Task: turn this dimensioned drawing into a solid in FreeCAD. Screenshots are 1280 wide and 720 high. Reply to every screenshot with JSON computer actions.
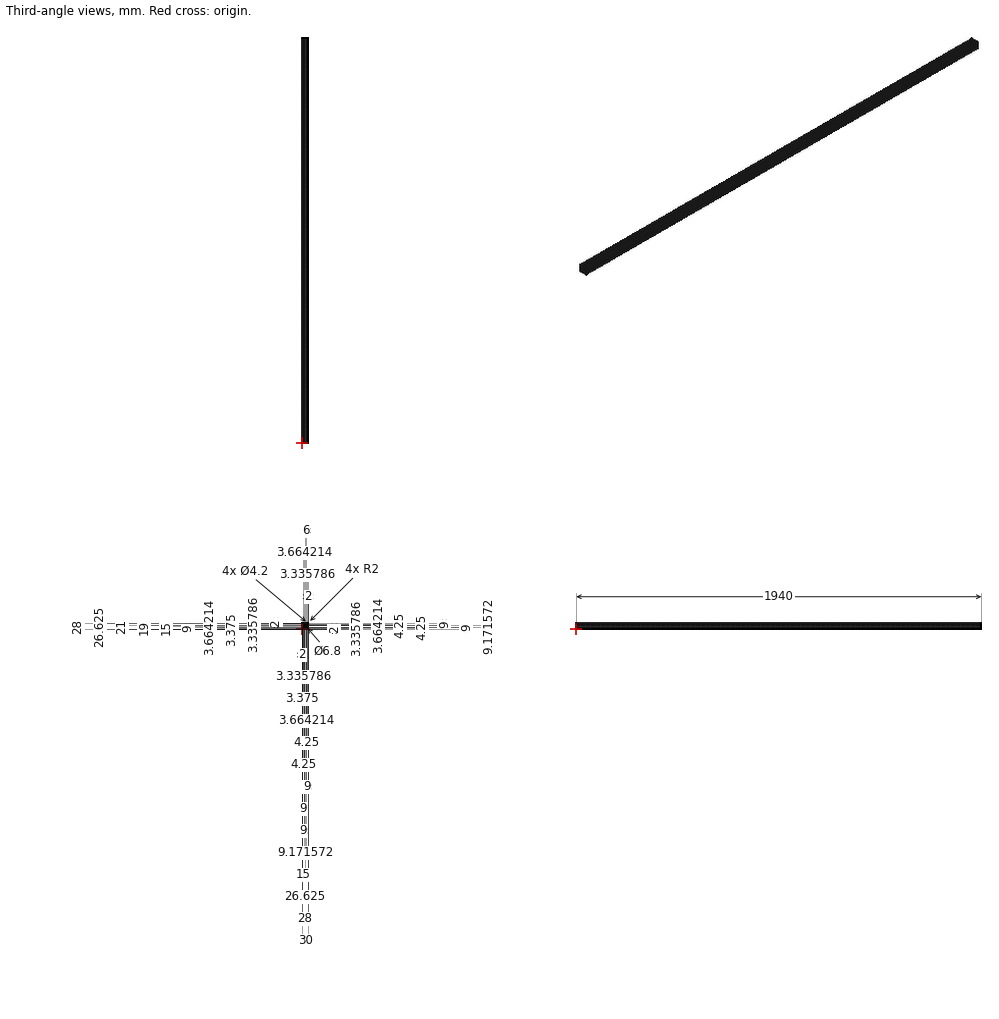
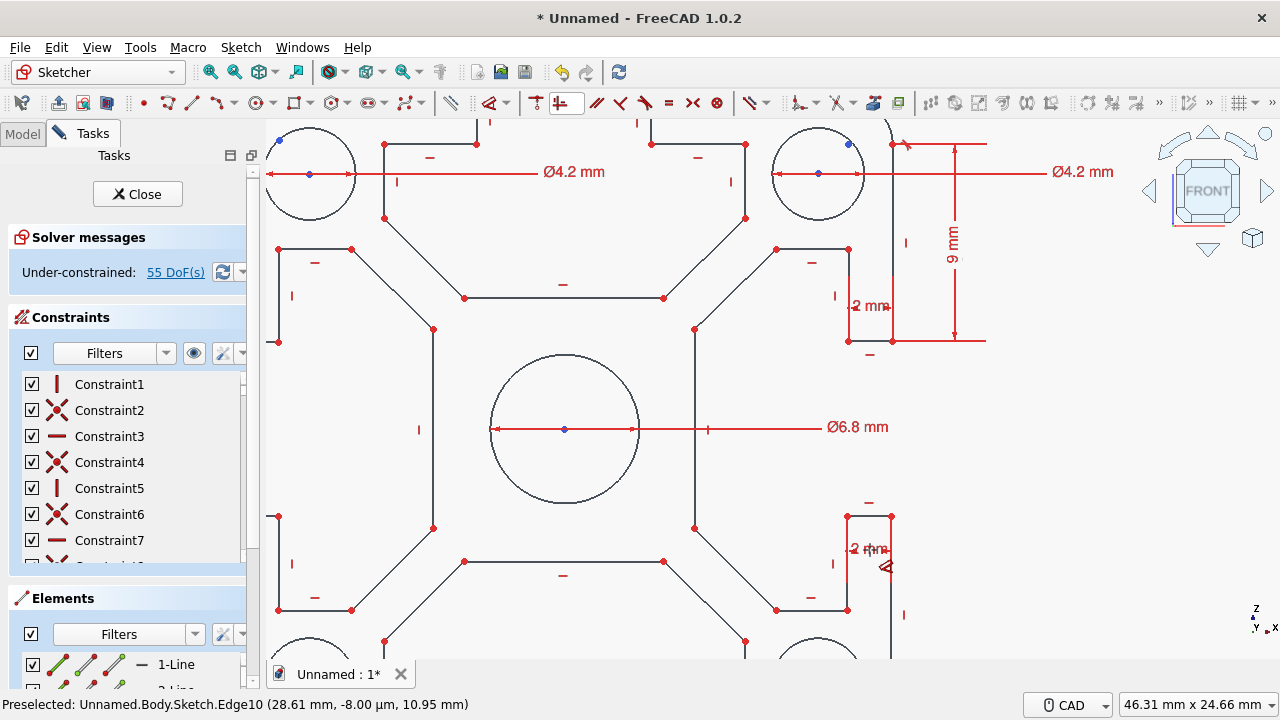
{"action": "left_click", "coordinate": [891, 575]}
{"action": "left_click", "coordinate": [925, 574]}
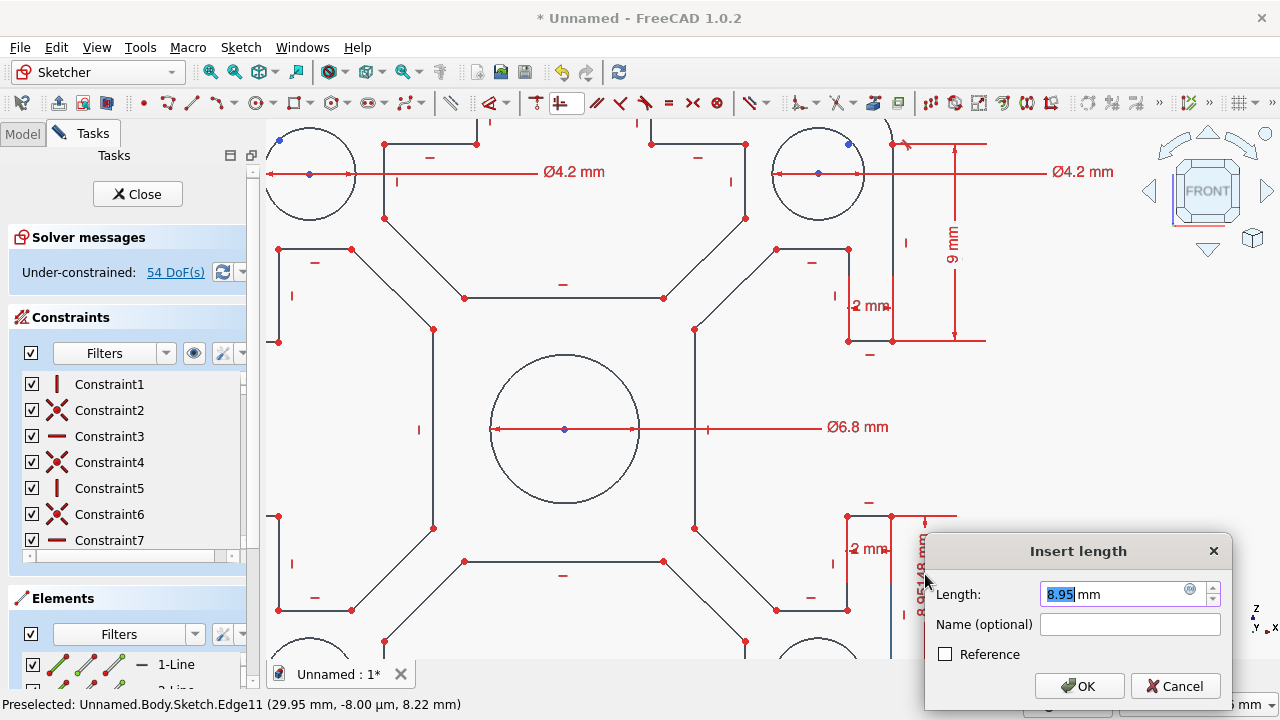
{"action": "type", "text": "9"}
{"action": "key", "text": "Return"}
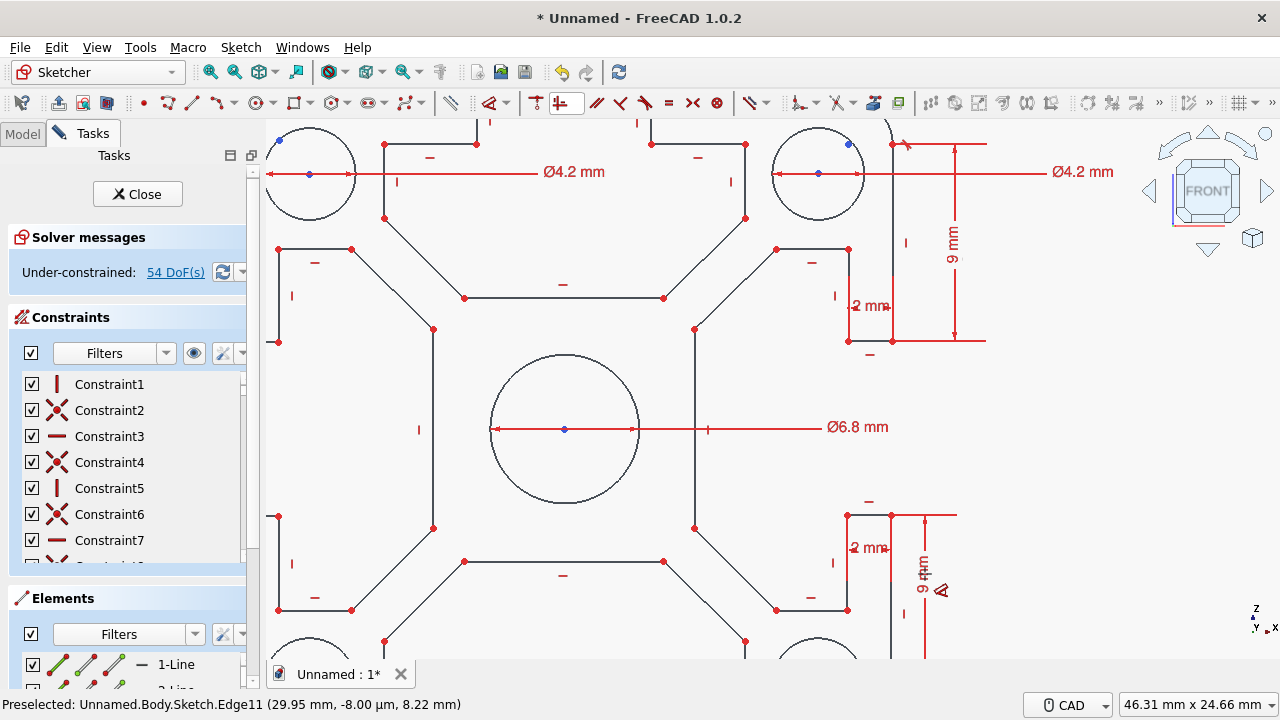
{"action": "scroll", "coordinate": [875, 342], "scroll_direction": "down", "scroll_amount": 3}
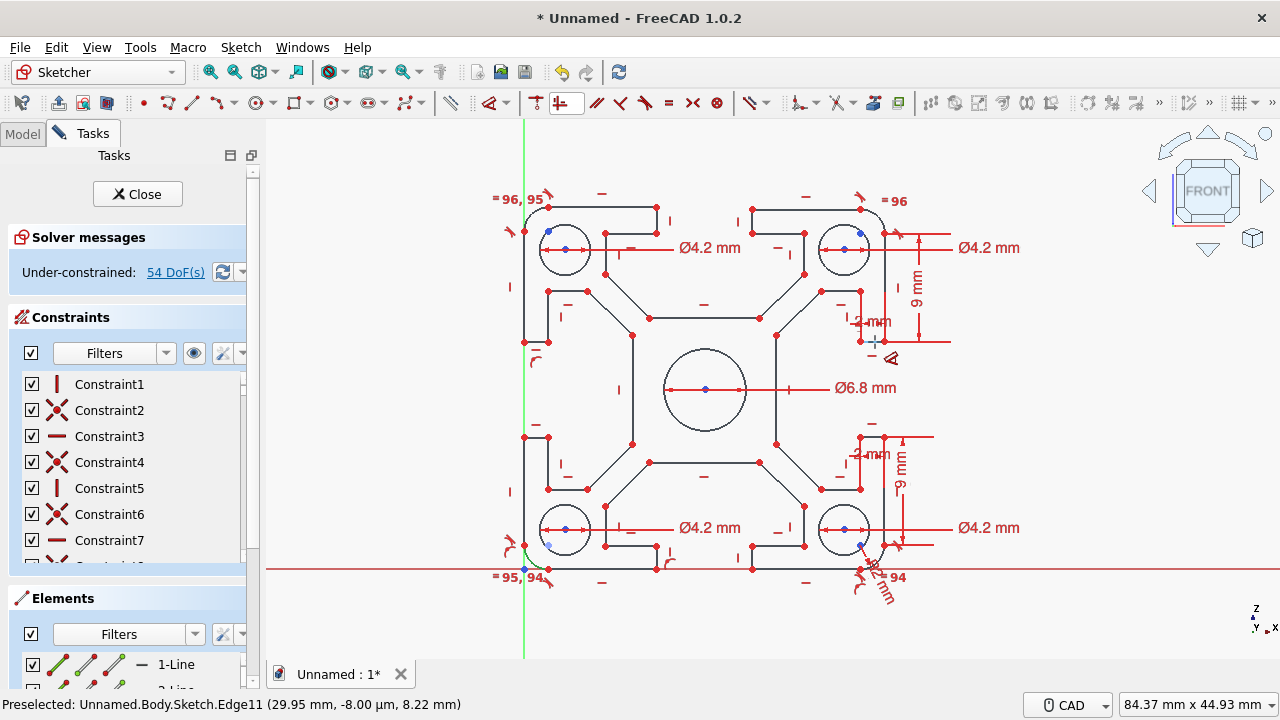
{"action": "left_click", "coordinate": [828, 569]}
{"action": "left_click", "coordinate": [806, 603]}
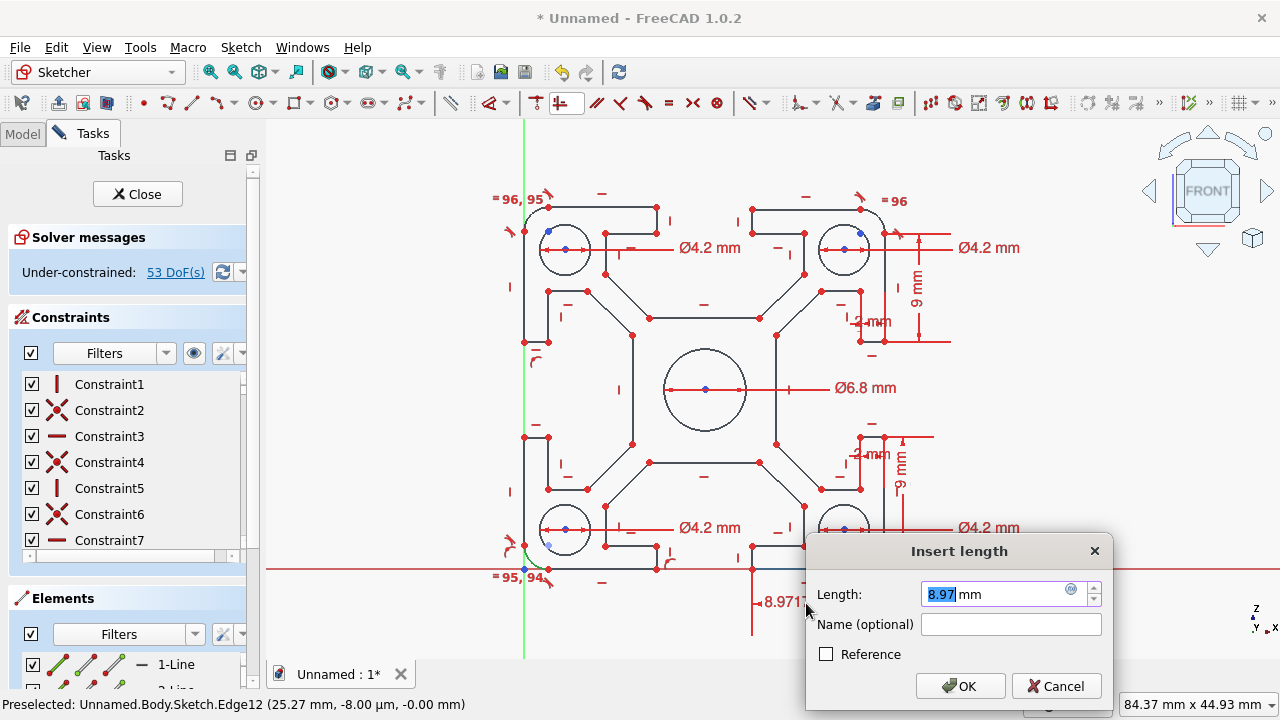
{"action": "type", "text": "9"}
{"action": "key", "text": "Return"}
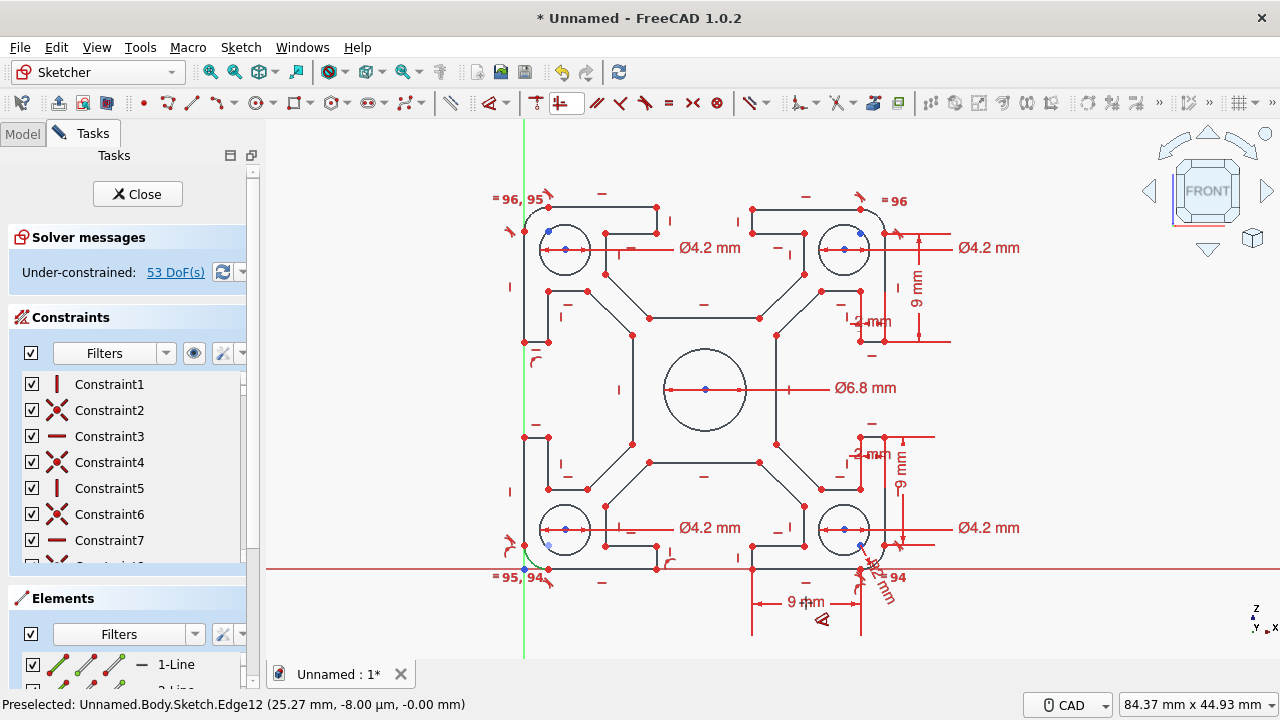
{"action": "scroll", "coordinate": [752, 560], "scroll_direction": "up", "scroll_amount": 3}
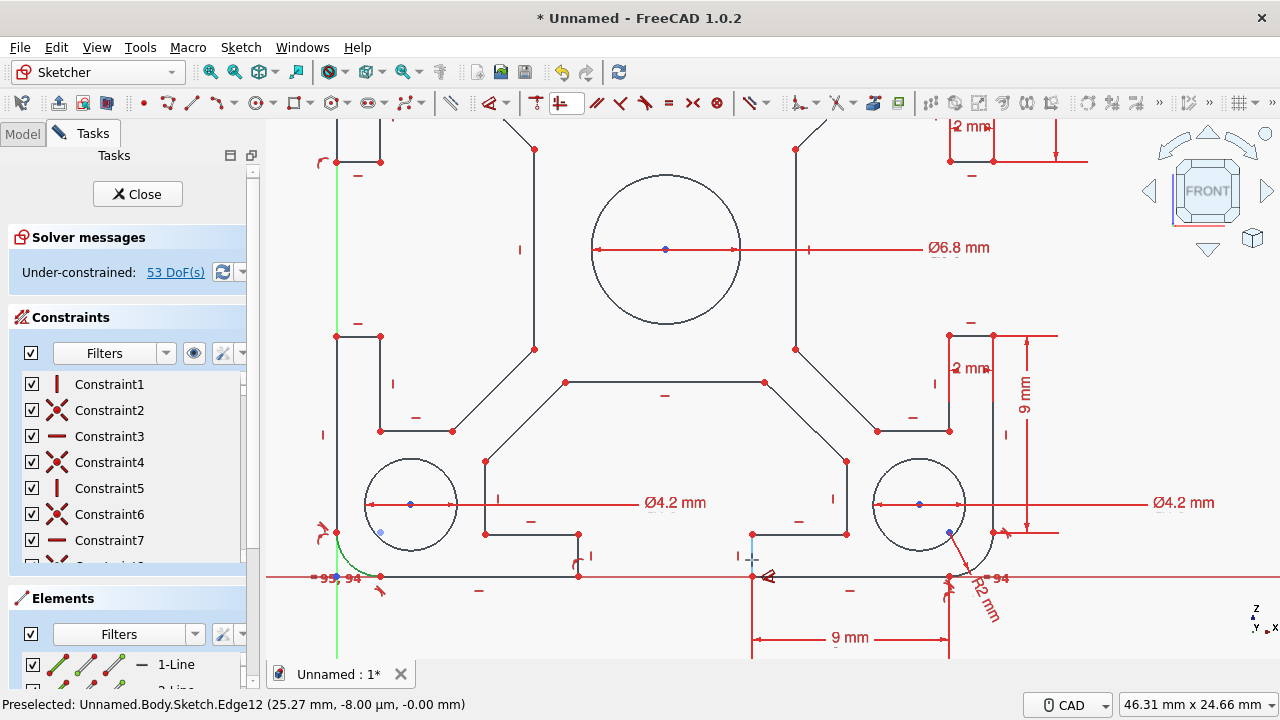
{"action": "left_click", "coordinate": [752, 560]}
{"action": "left_click", "coordinate": [786, 556]}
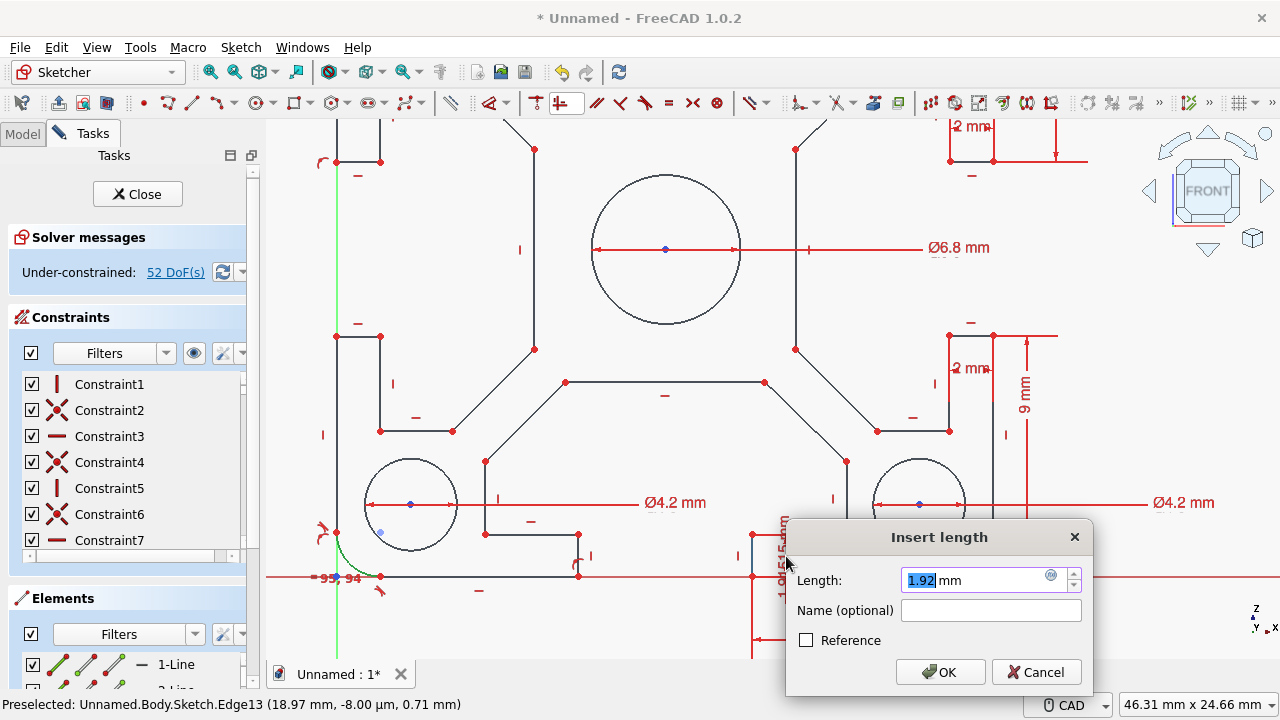
{"action": "type", "text": "2"}
{"action": "key", "text": "Return"}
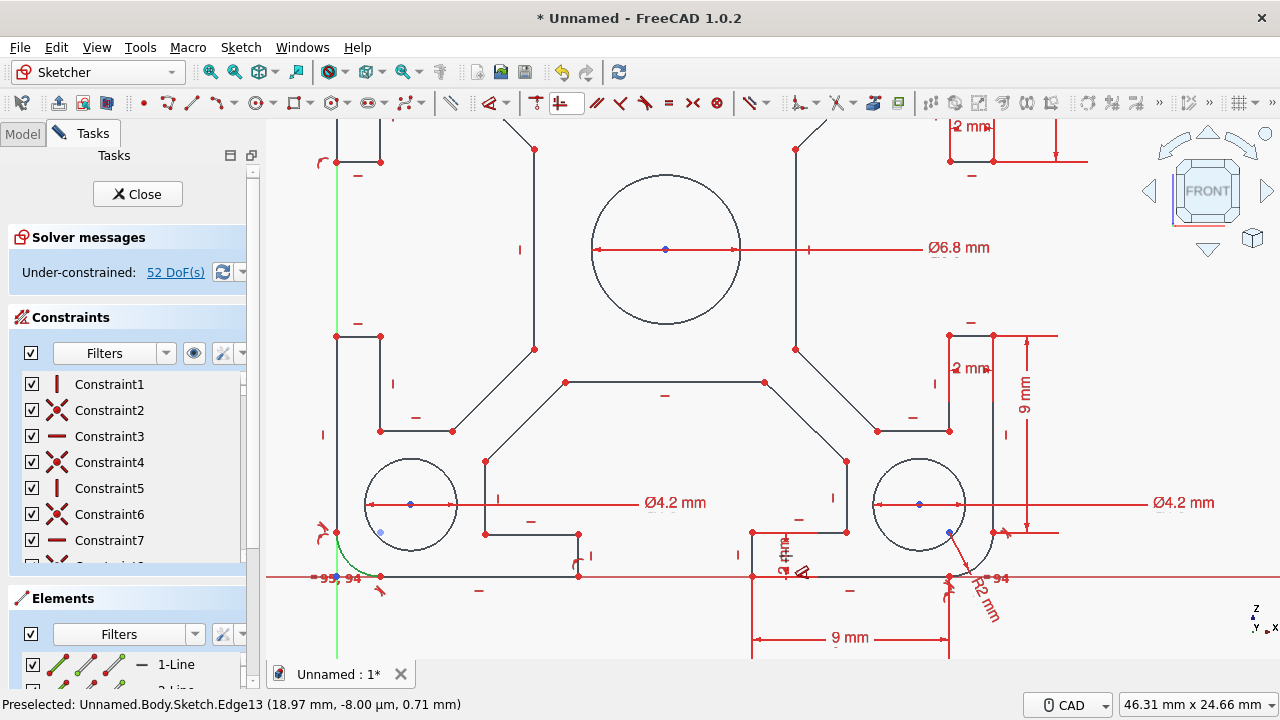
{"action": "left_click", "coordinate": [578, 547]}
{"action": "left_click", "coordinate": [544, 556]}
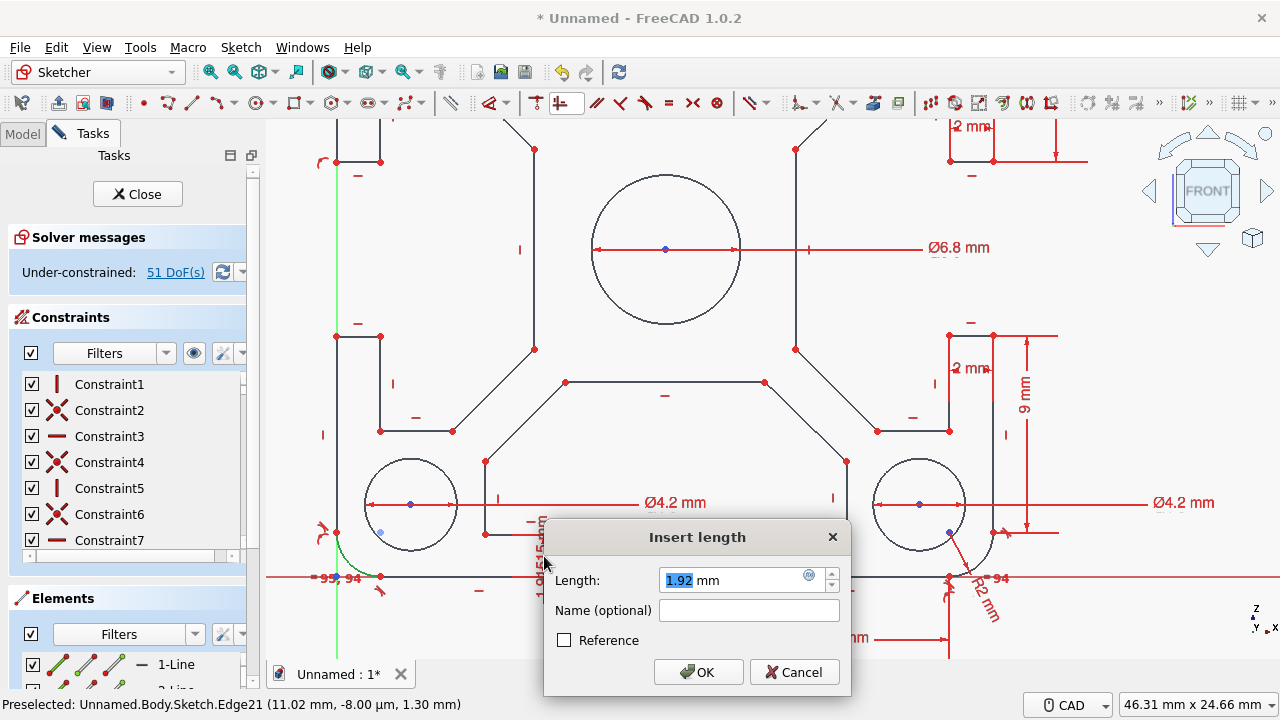
{"action": "type", "text": "2"}
{"action": "key", "text": "Return"}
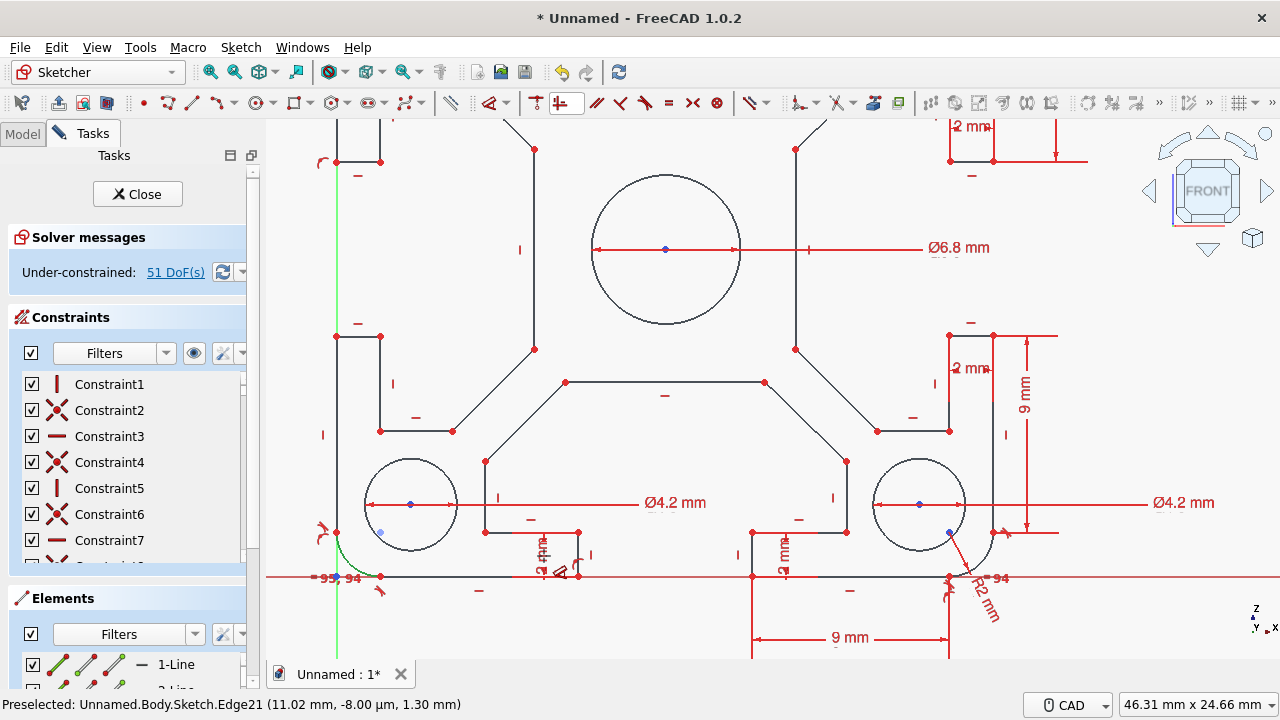
{"action": "left_click", "coordinate": [519, 577]}
{"action": "left_click", "coordinate": [479, 611]}